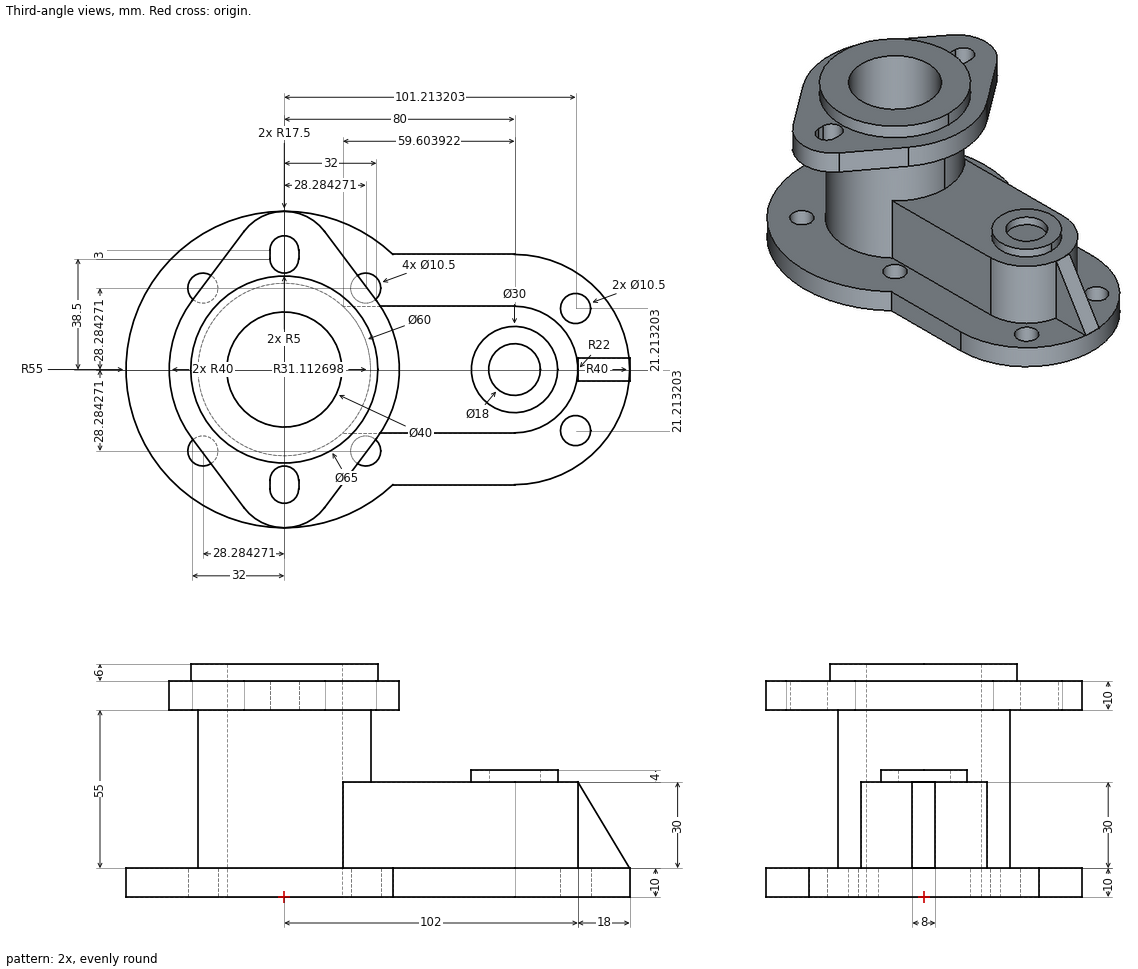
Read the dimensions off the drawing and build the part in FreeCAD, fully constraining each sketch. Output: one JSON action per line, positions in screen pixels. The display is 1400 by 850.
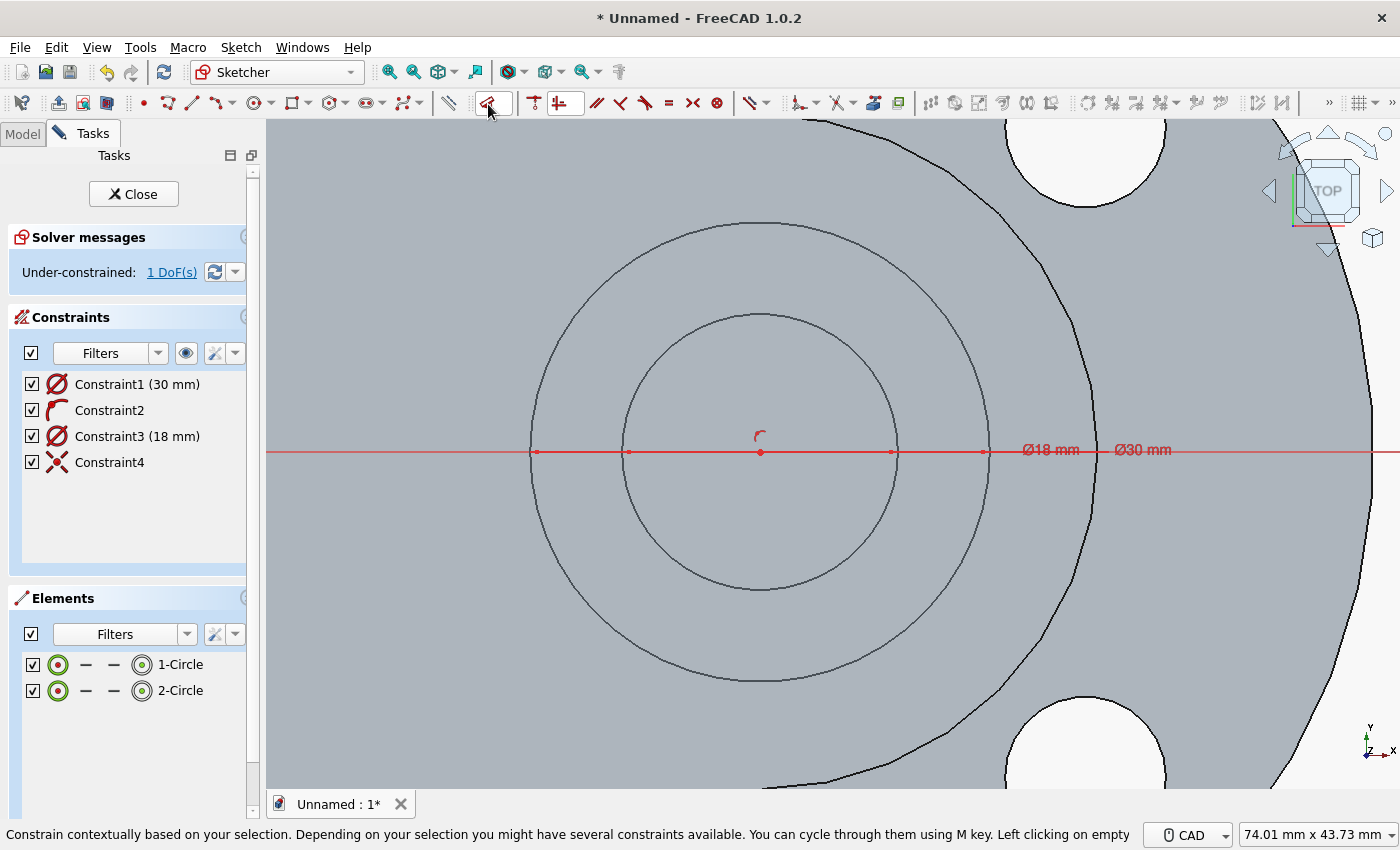
{"action": "left_click", "coordinate": [760, 452]}
{"action": "left_click", "coordinate": [420, 486]}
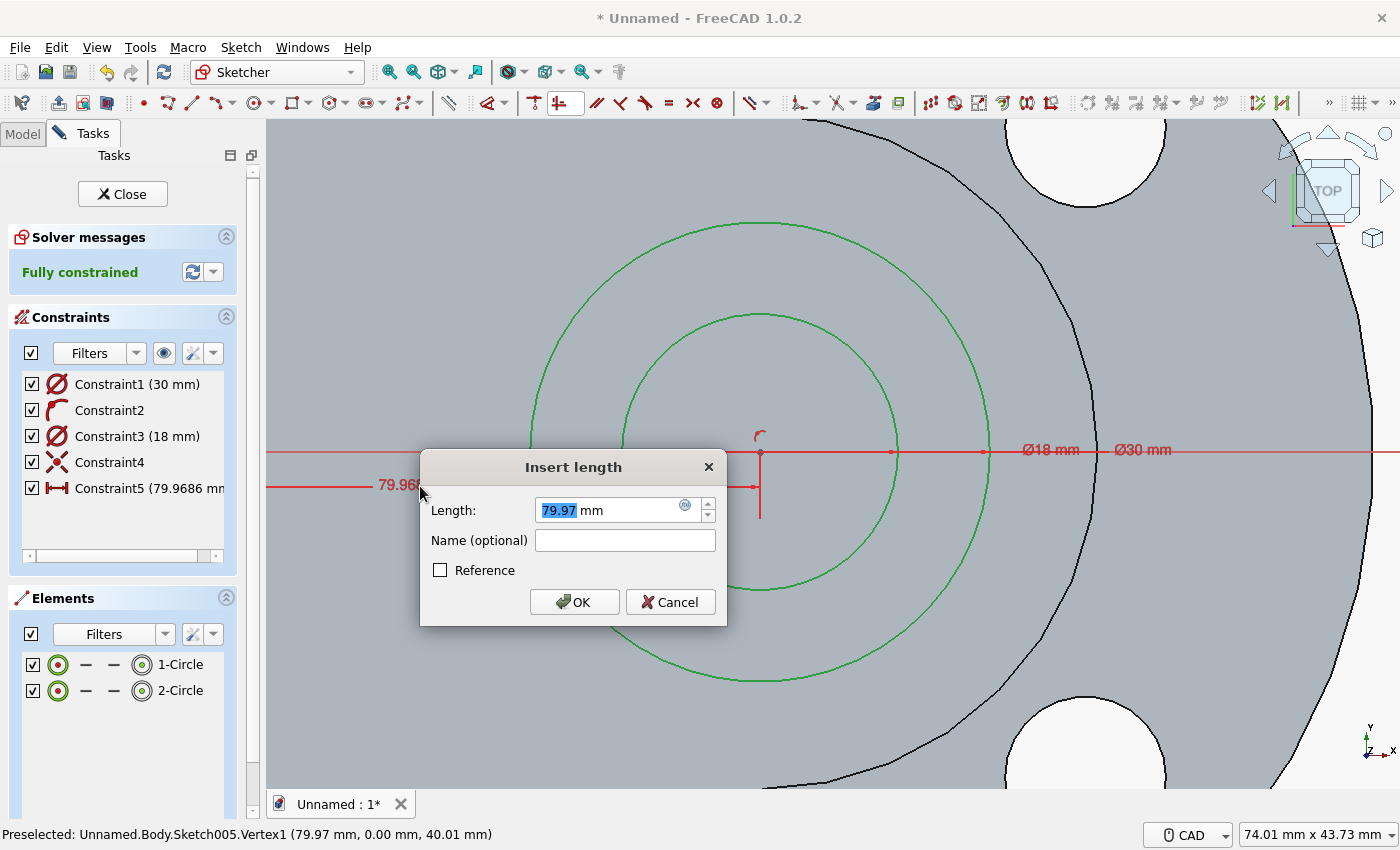
{"action": "type", "text": "80"}
{"action": "key", "text": "Return"}
{"action": "key", "text": "Escape"}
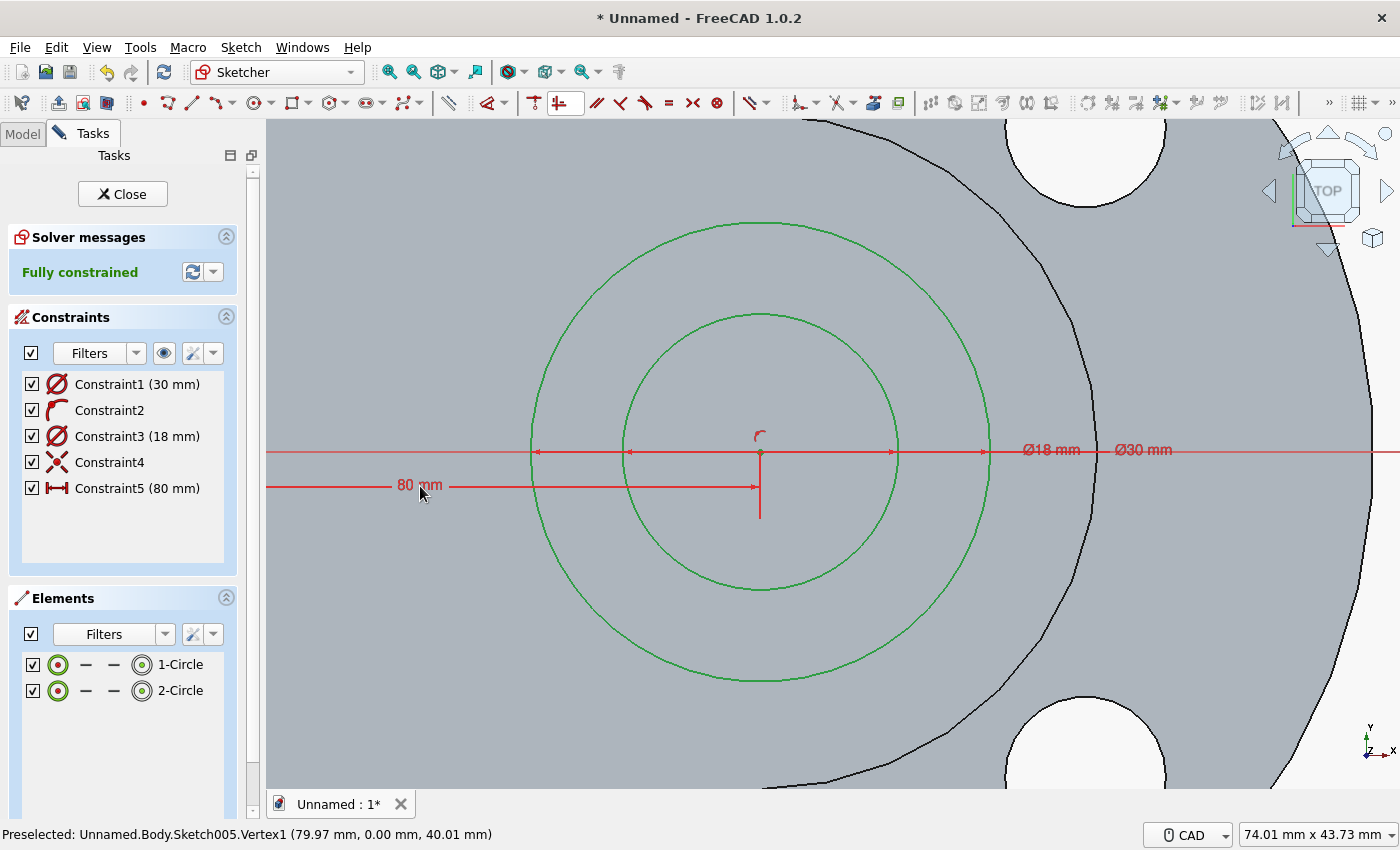
{"action": "left_click", "coordinate": [123, 194]}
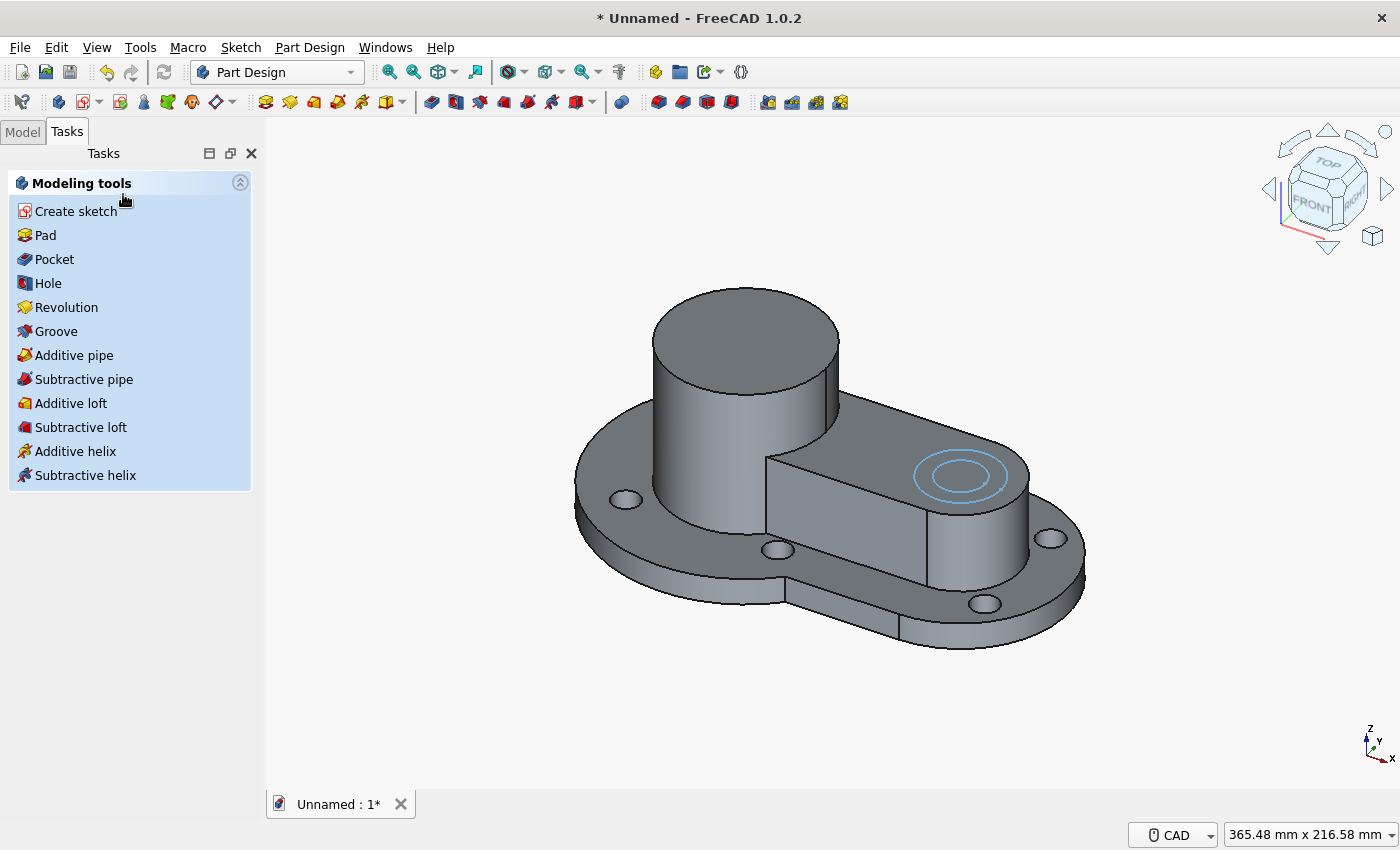
{"action": "left_click", "coordinate": [266, 102]}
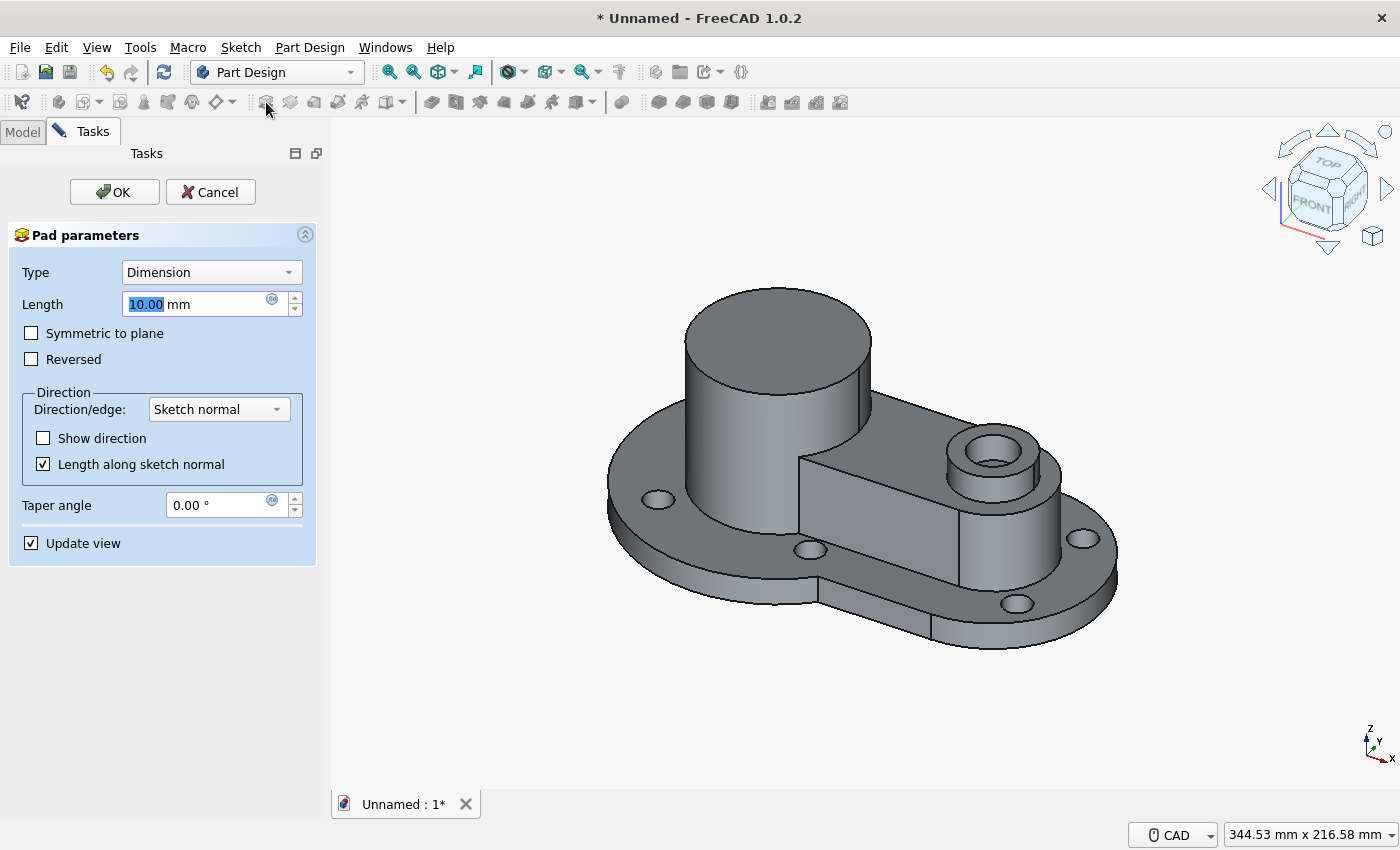
{"action": "type", "text": "4"}
{"action": "key", "text": "Tab"}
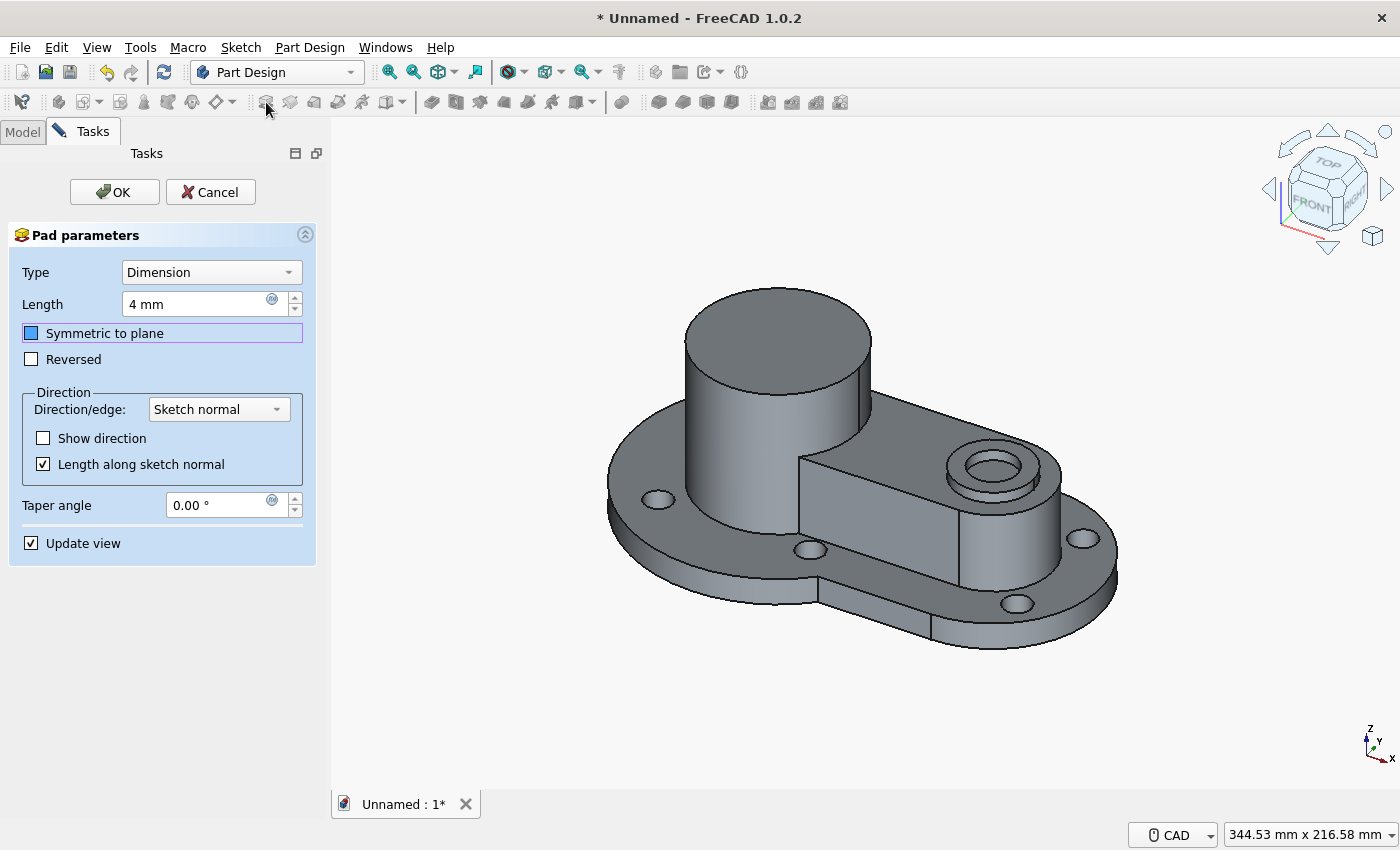
{"action": "left_click", "coordinate": [115, 192]}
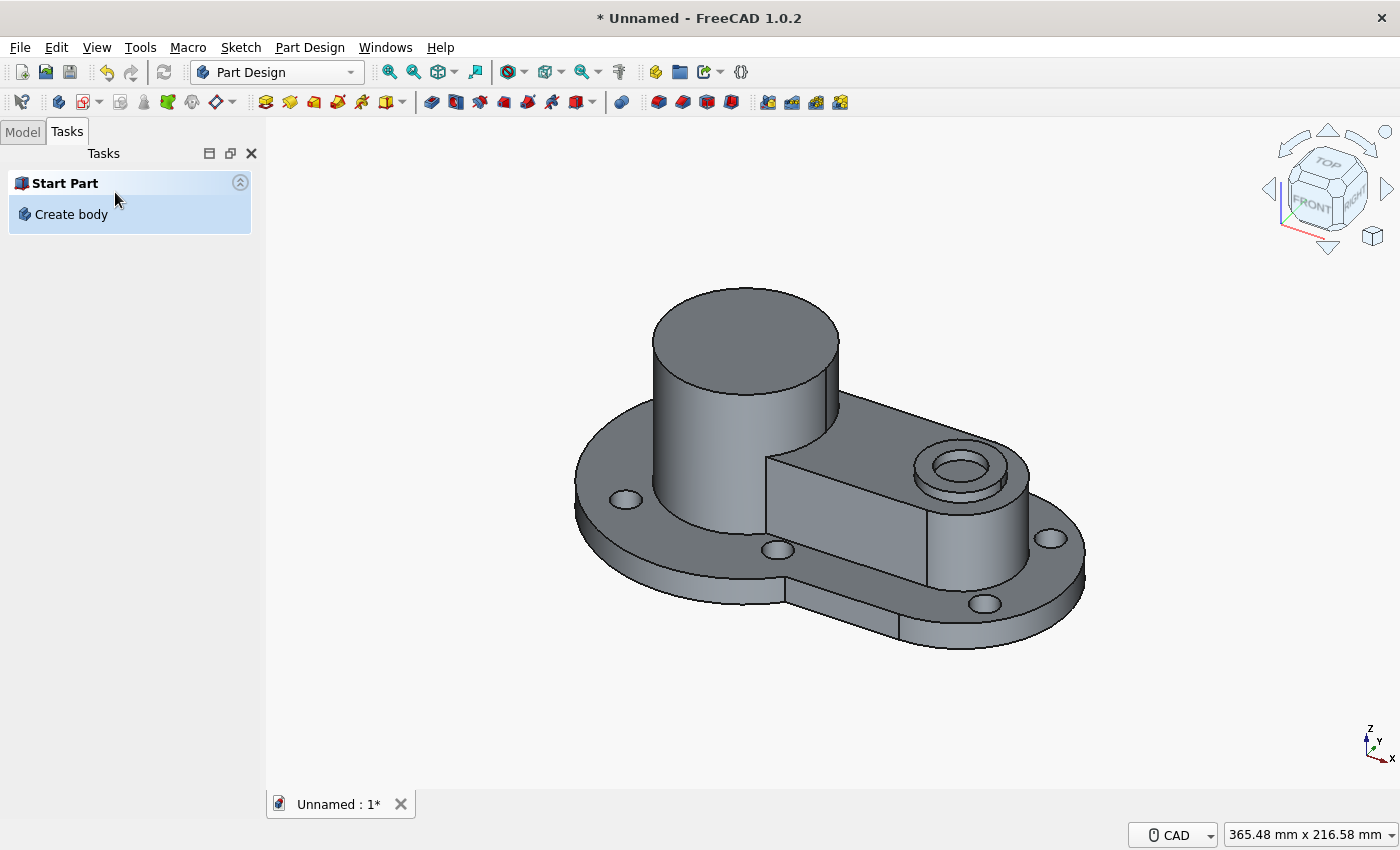
{"action": "left_click", "coordinate": [746, 341]}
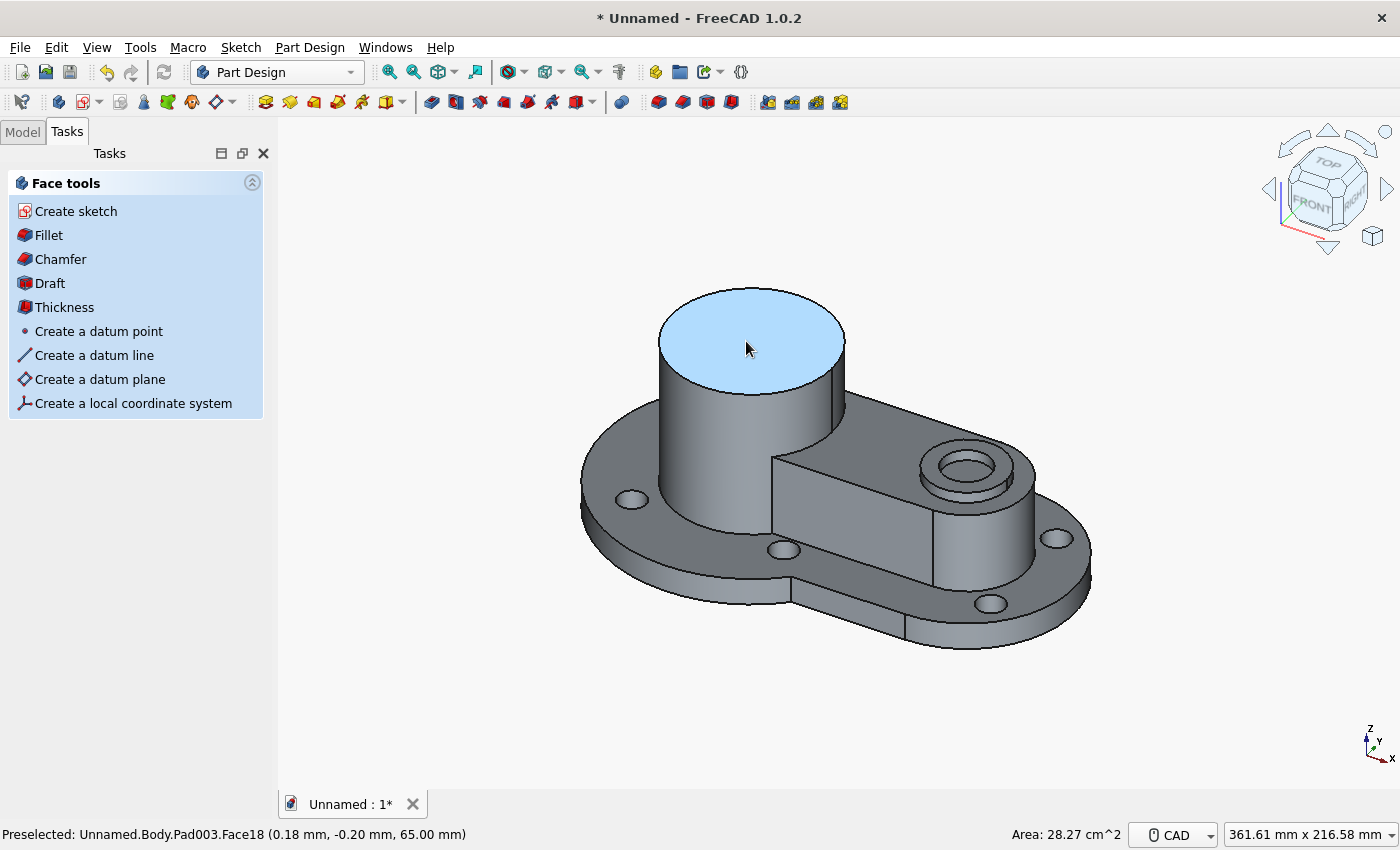
{"action": "left_click", "coordinate": [84, 102]}